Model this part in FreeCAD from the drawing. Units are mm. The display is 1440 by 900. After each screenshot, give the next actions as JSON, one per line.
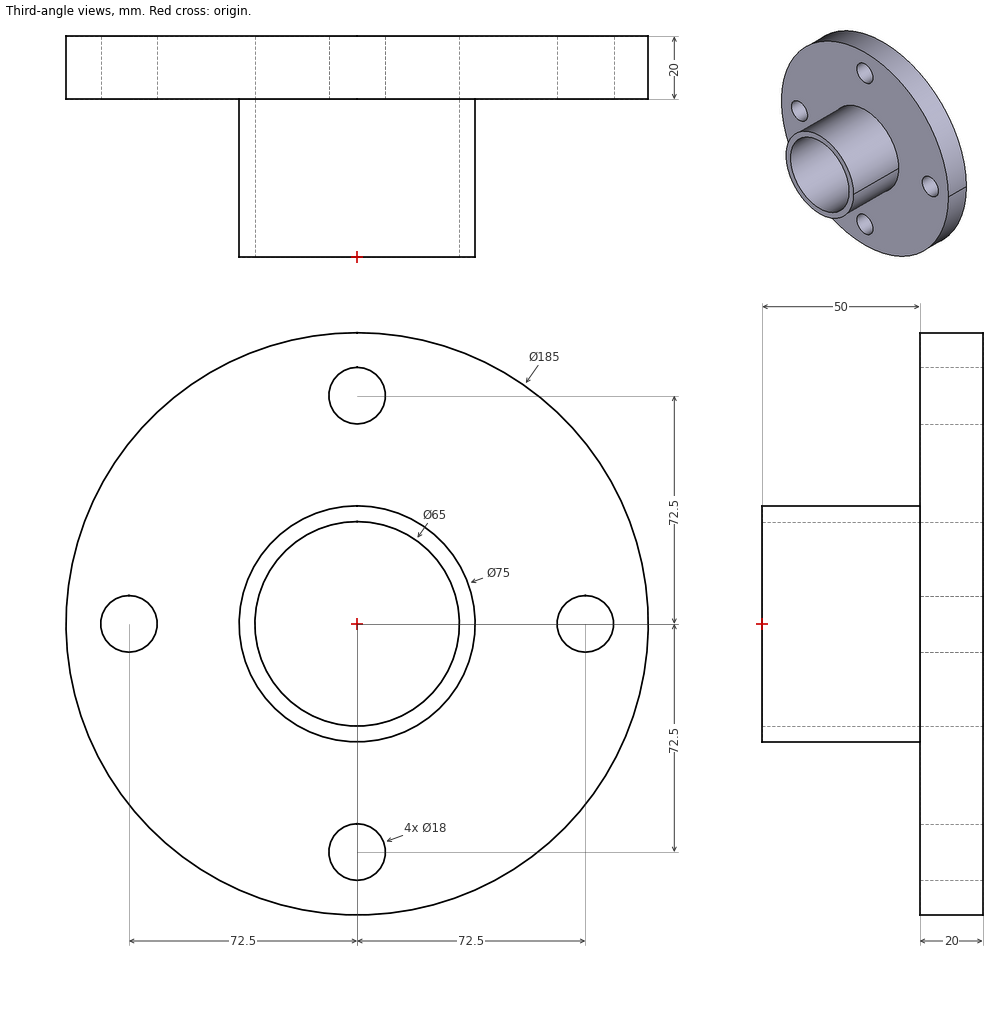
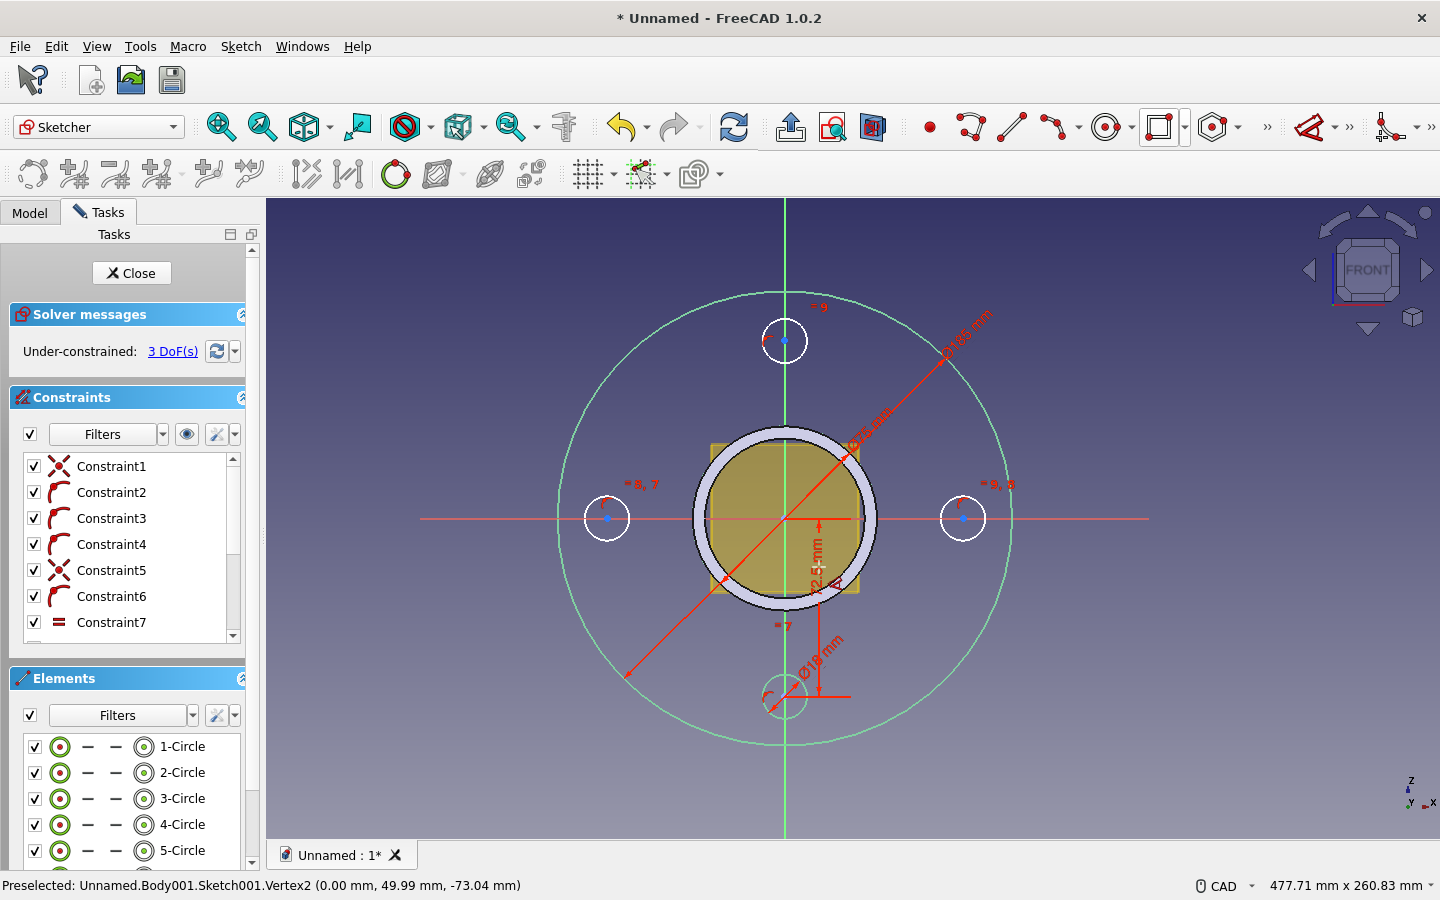
{"action": "left_click", "coordinate": [607, 519]}
{"action": "left_click", "coordinate": [655, 553]}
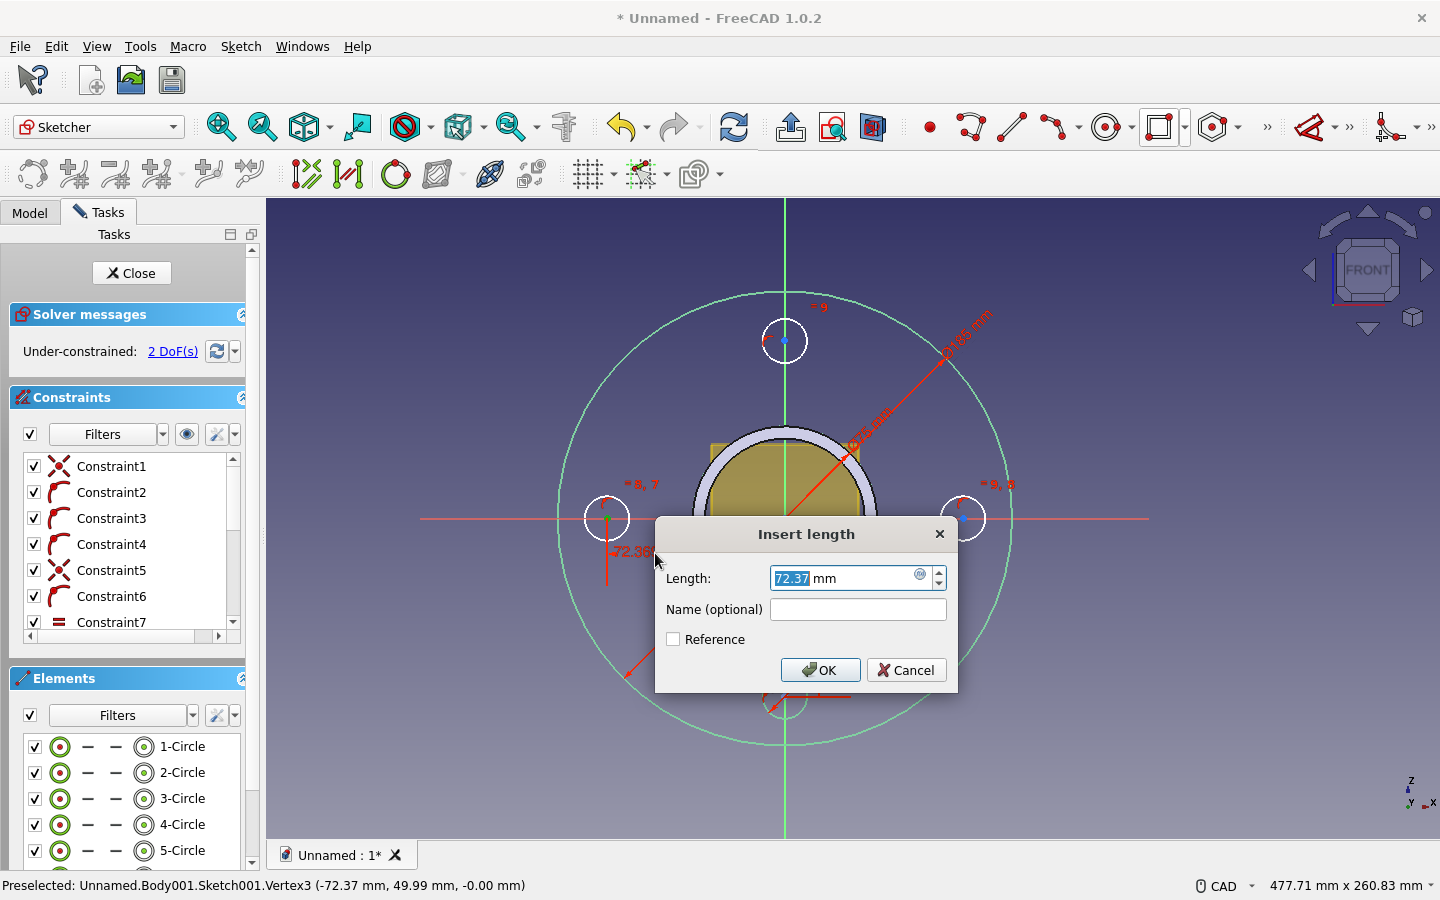
{"action": "type", "text": "72.5"}
{"action": "key", "text": "Return"}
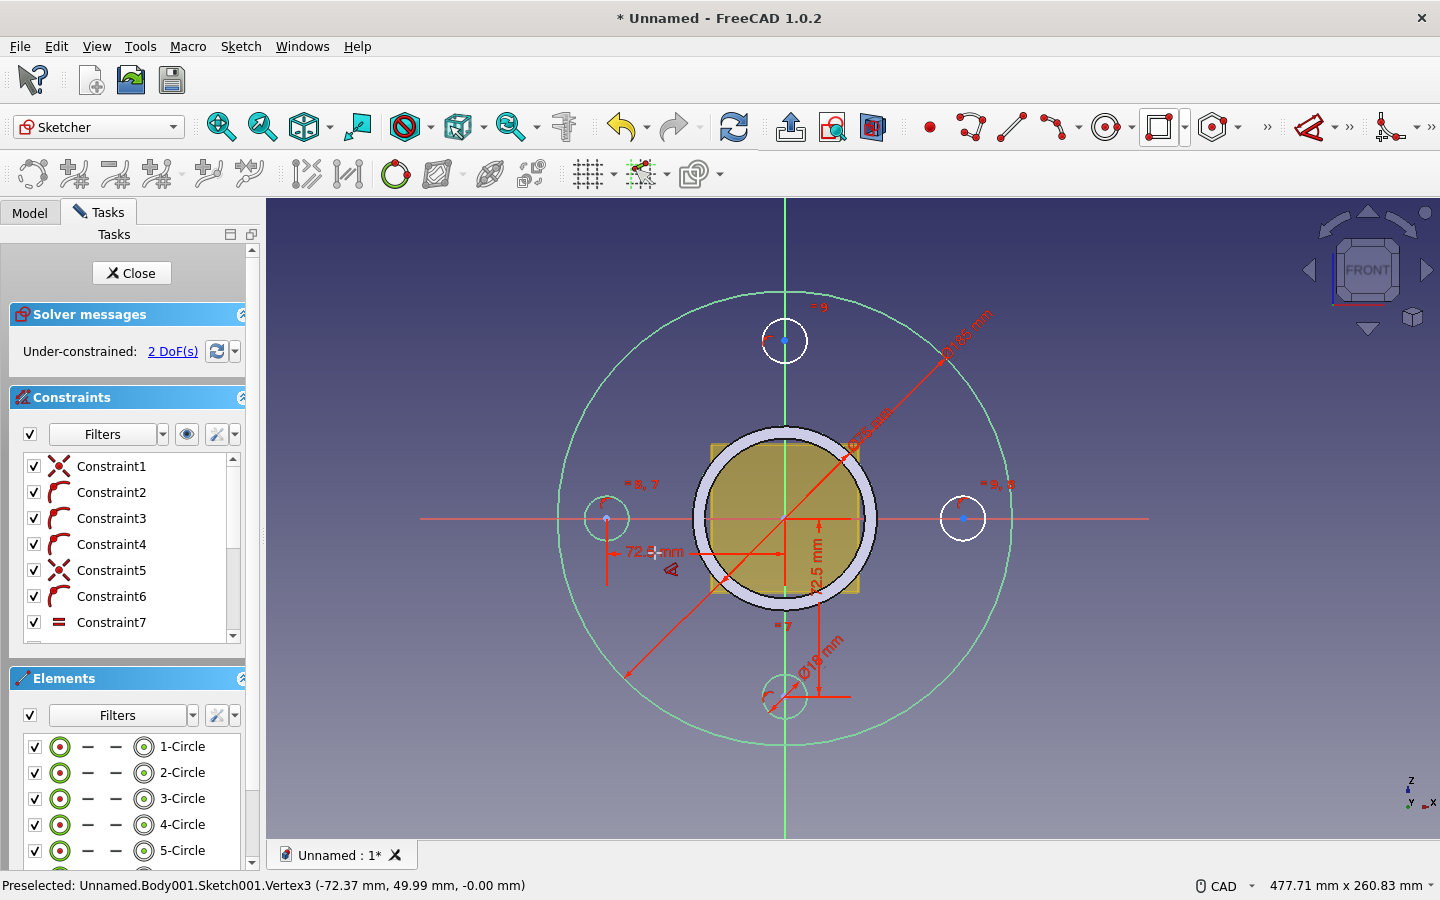
{"action": "left_click", "coordinate": [963, 519]}
{"action": "left_click", "coordinate": [915, 553]}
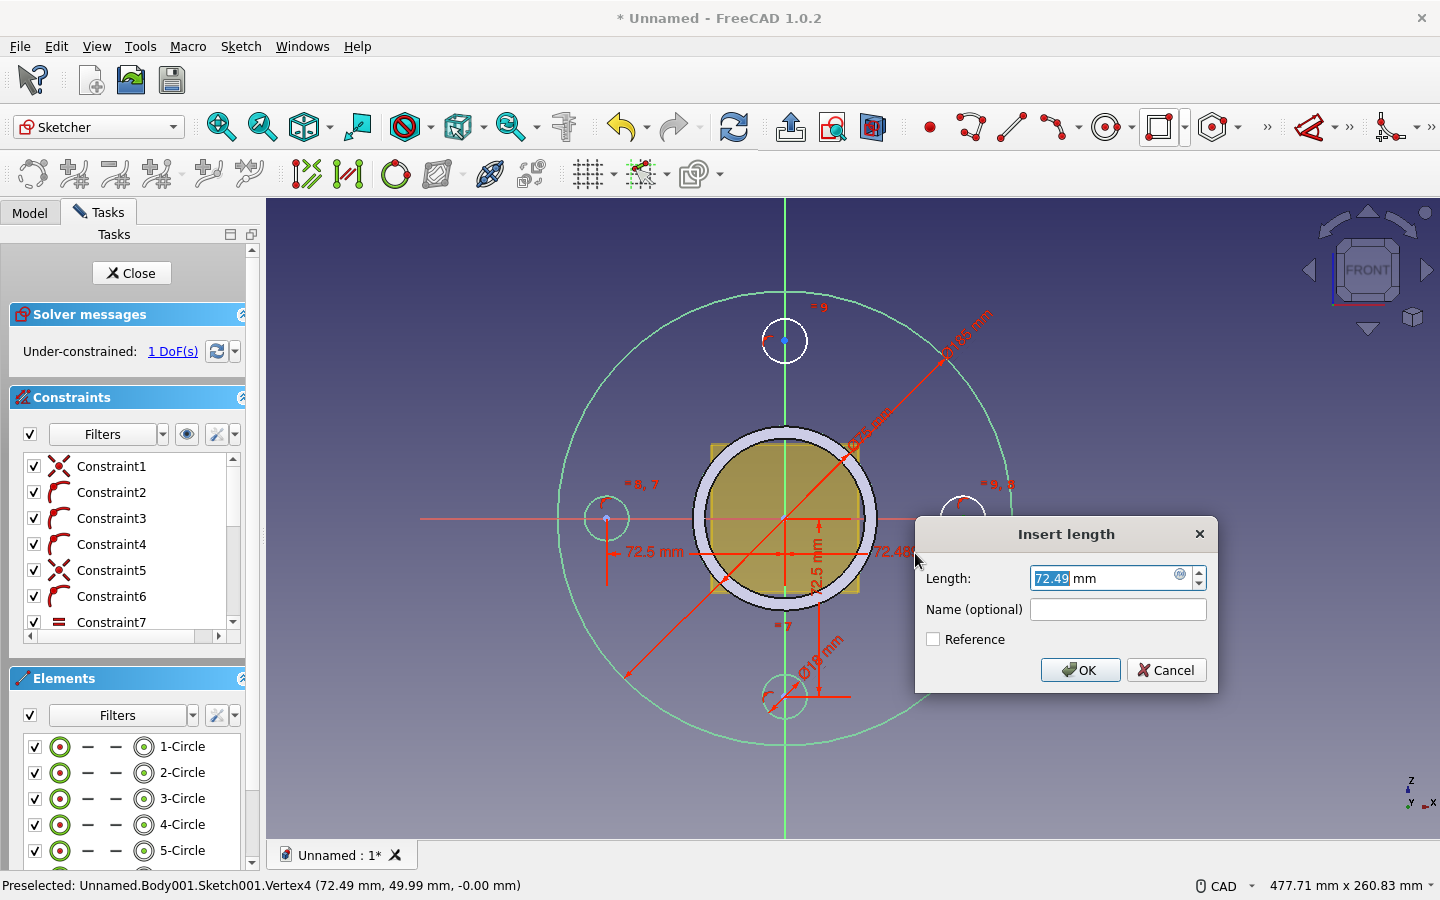
{"action": "type", "text": "72.5"}
{"action": "key", "text": "Return"}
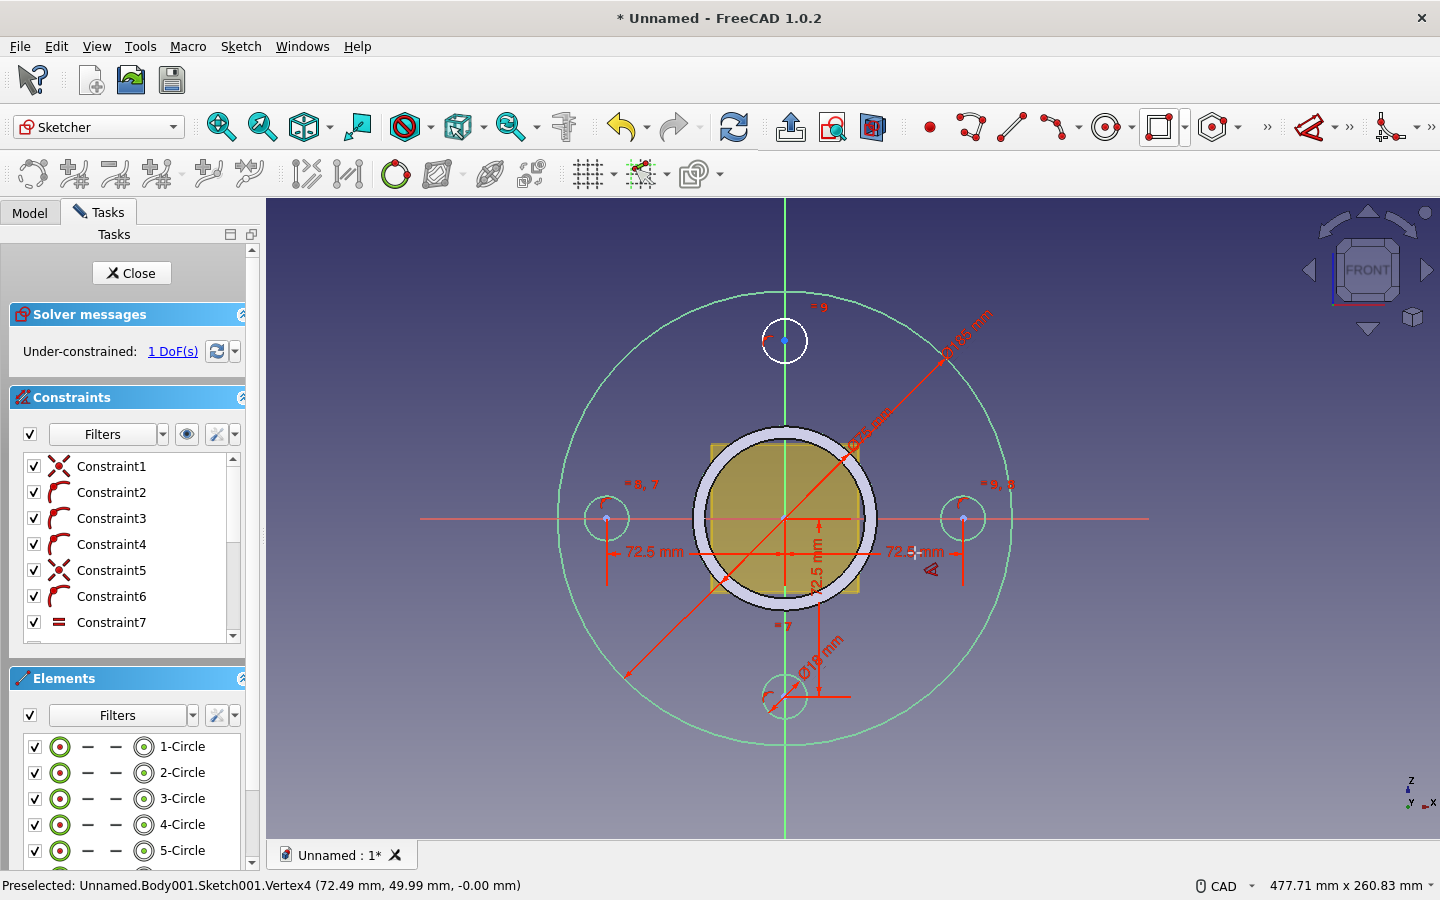
{"action": "left_click", "coordinate": [785, 341]}
{"action": "left_click", "coordinate": [819, 389]}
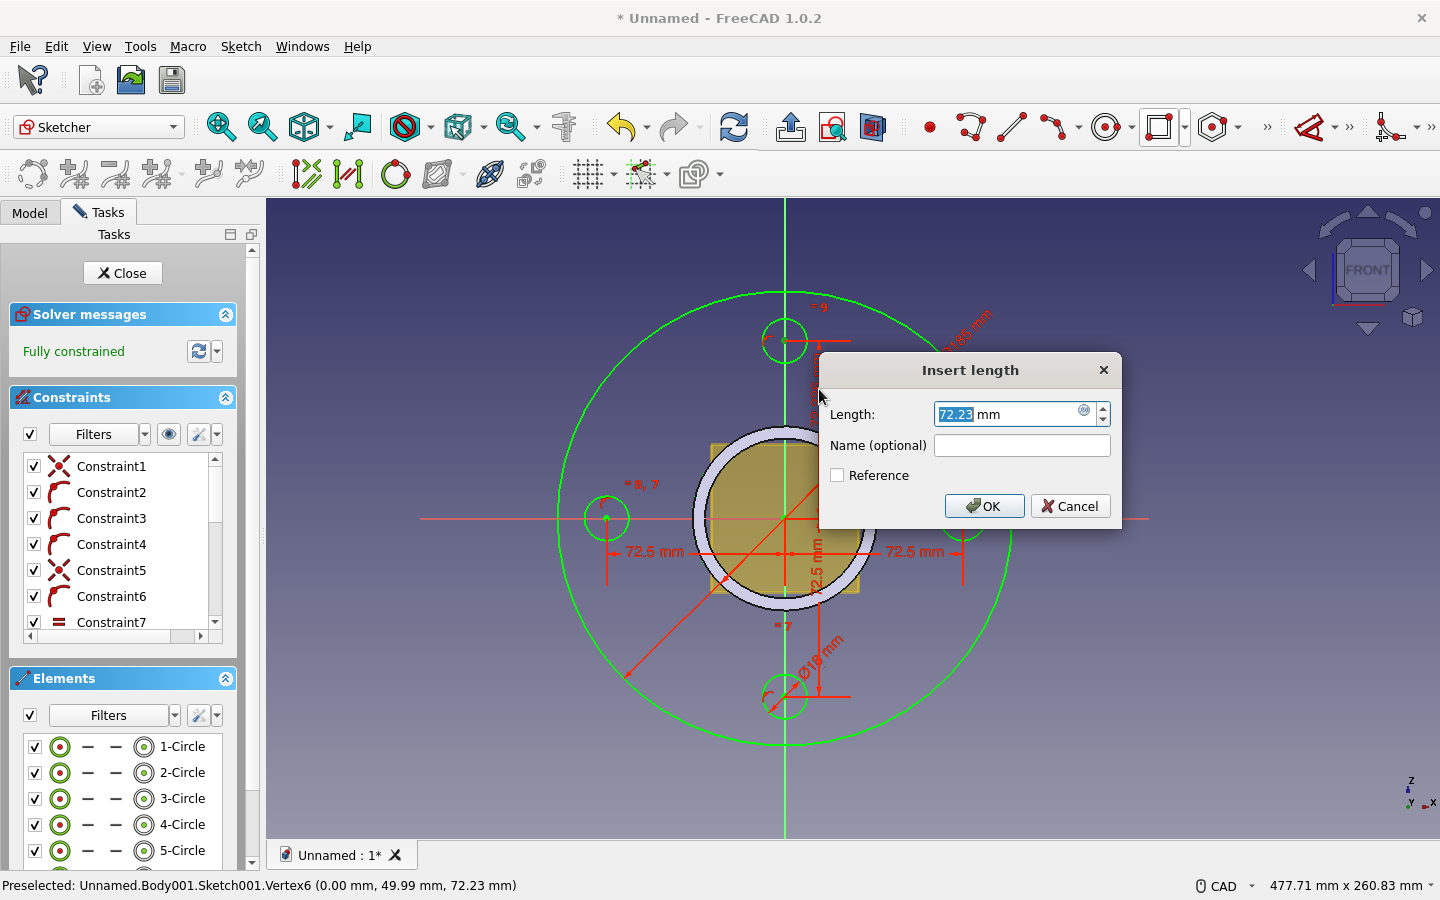
{"action": "type", "text": "72.5"}
{"action": "key", "text": "Return"}
{"action": "key", "text": "Escape"}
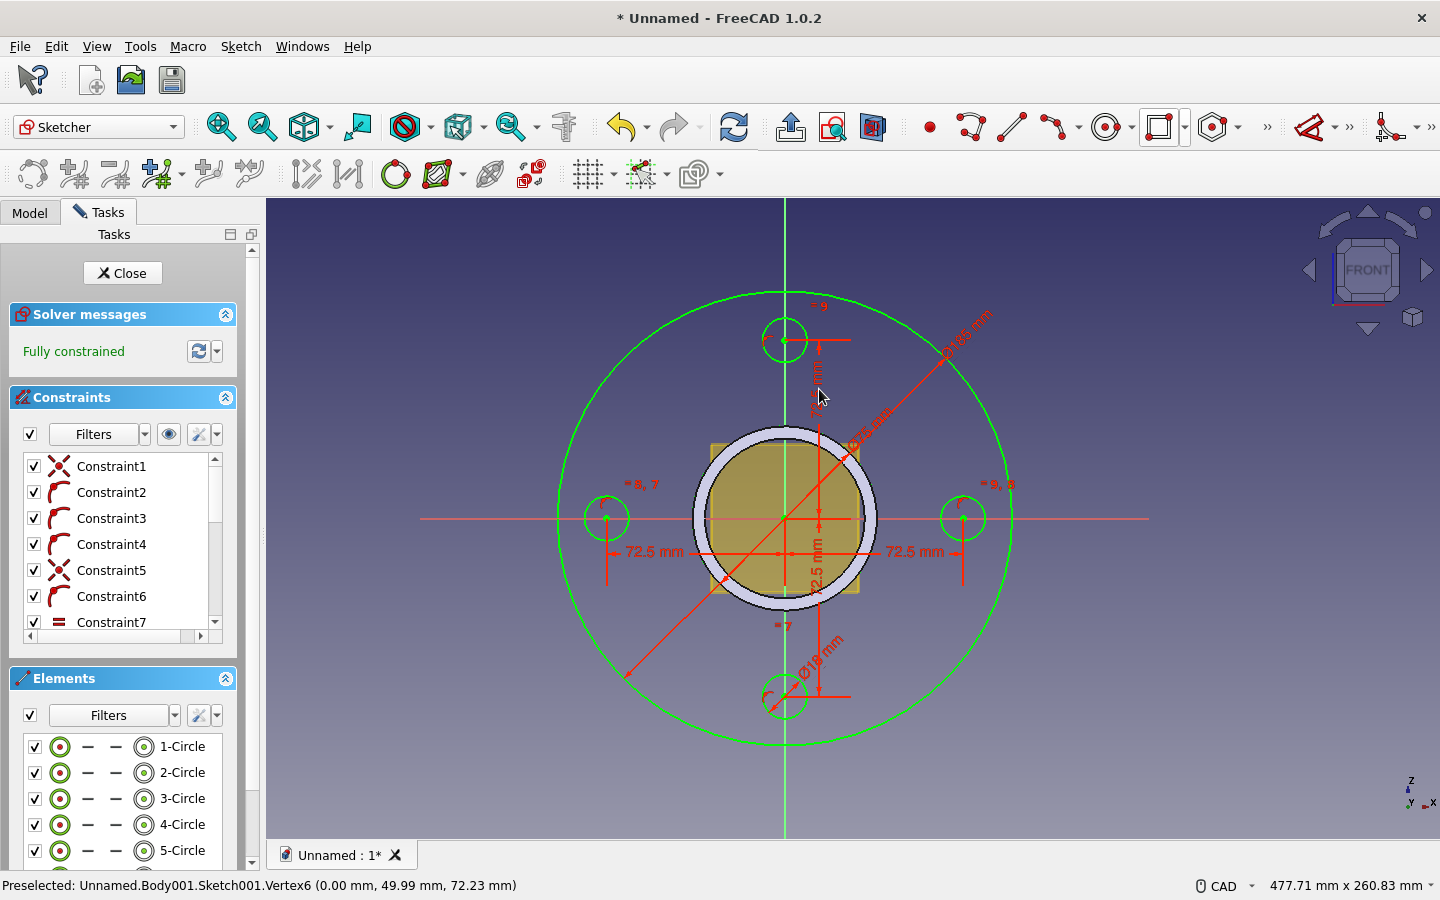
{"action": "left_click", "coordinate": [123, 273]}